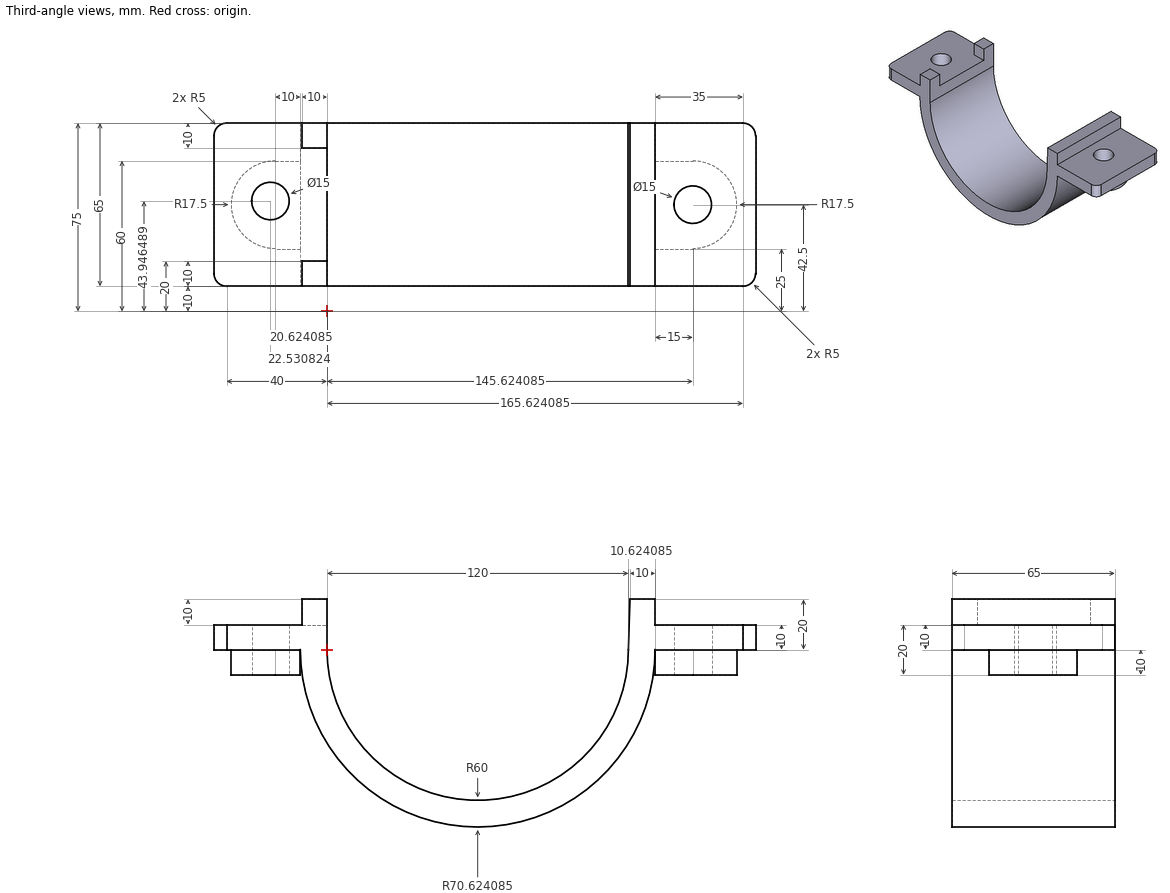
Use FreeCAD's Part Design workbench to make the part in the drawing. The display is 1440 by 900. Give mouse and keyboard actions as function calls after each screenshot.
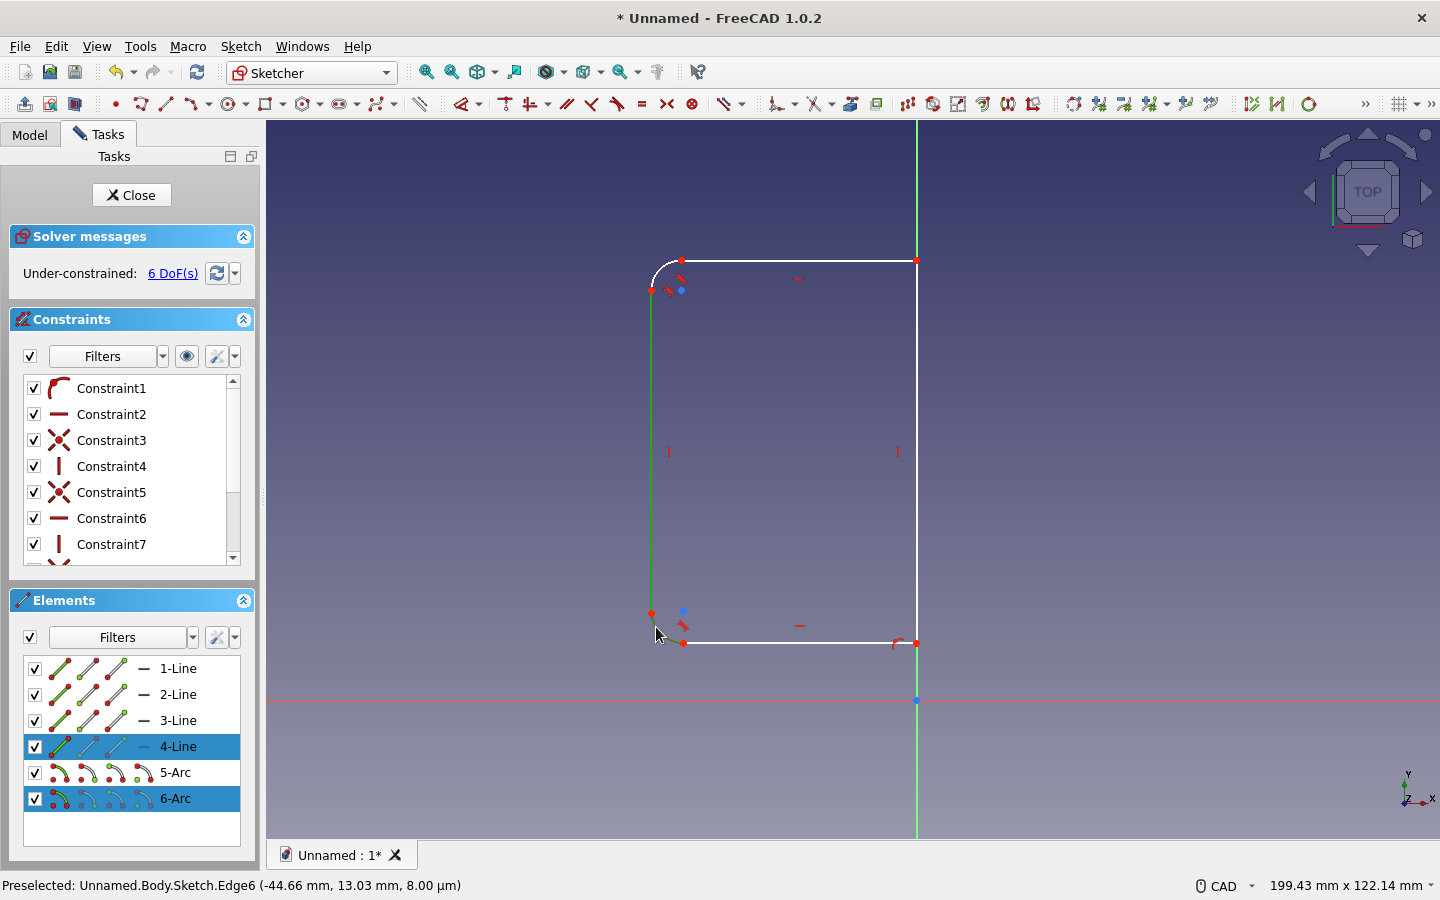
click(617, 104)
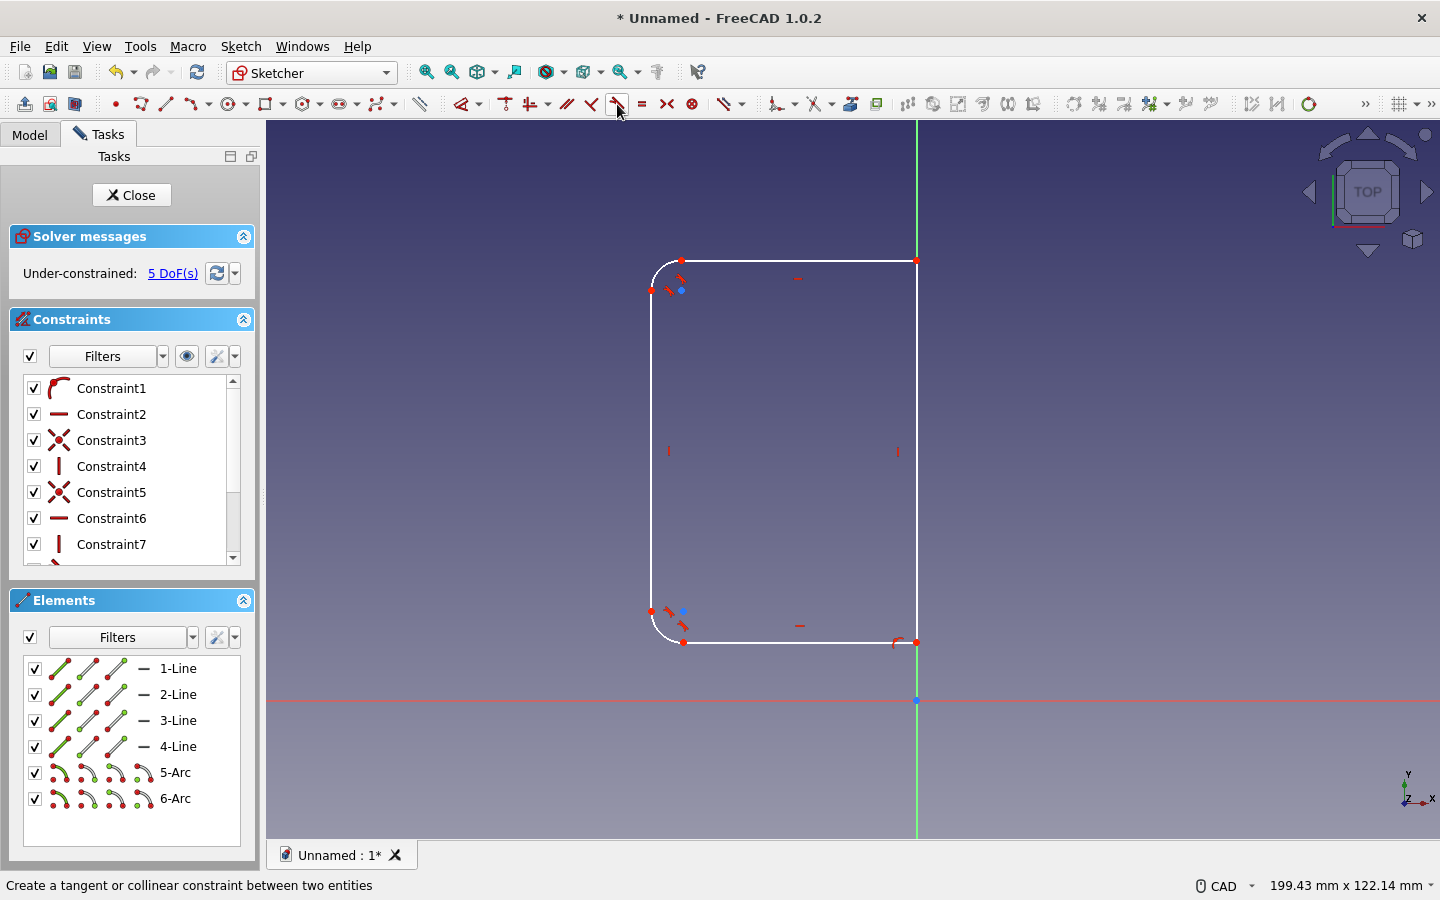
click(668, 264)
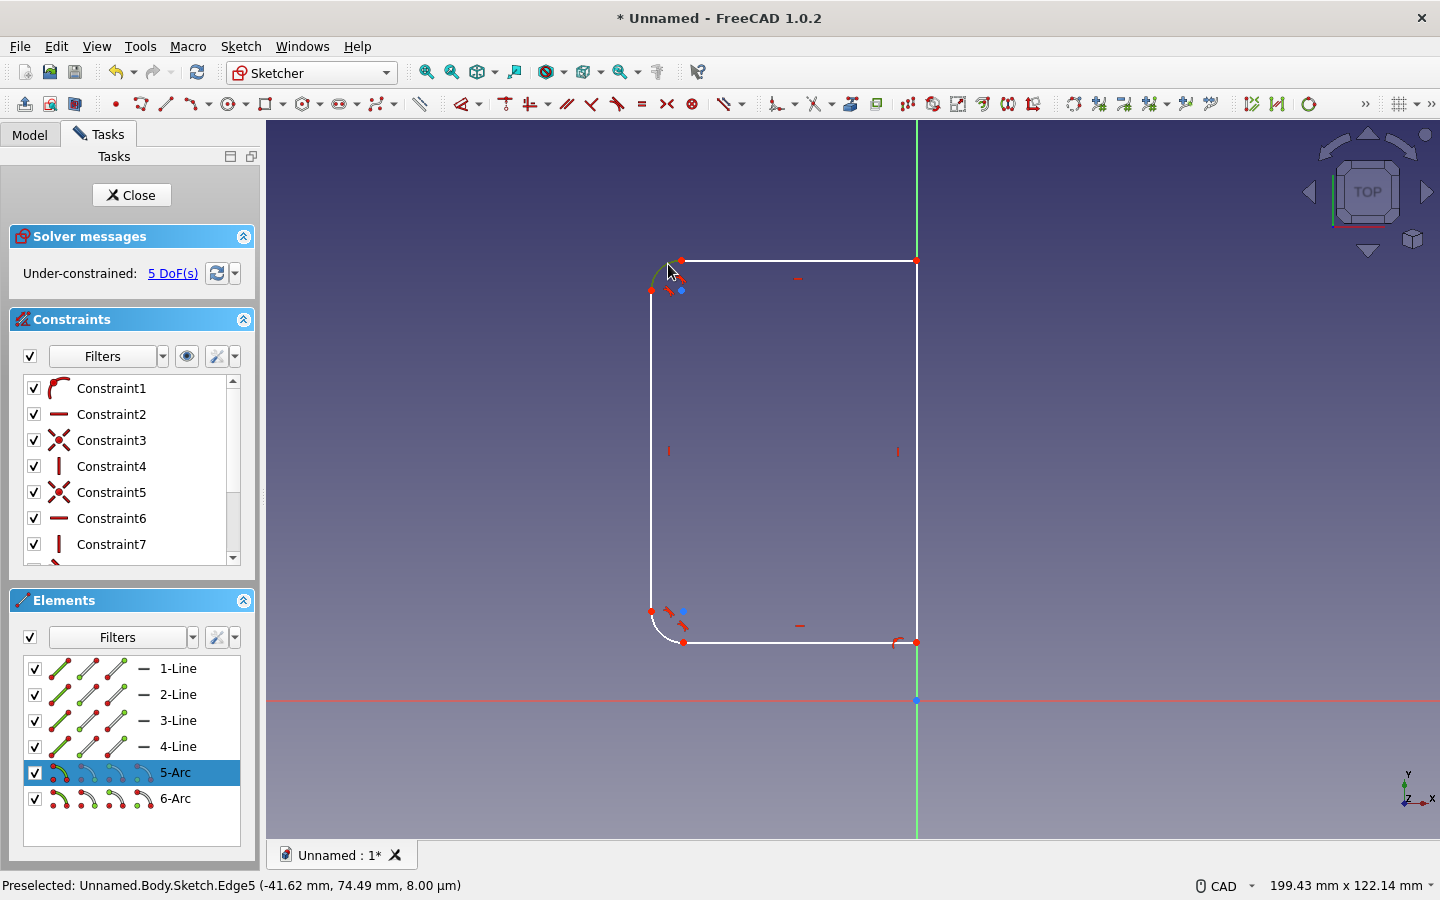
click(655, 626)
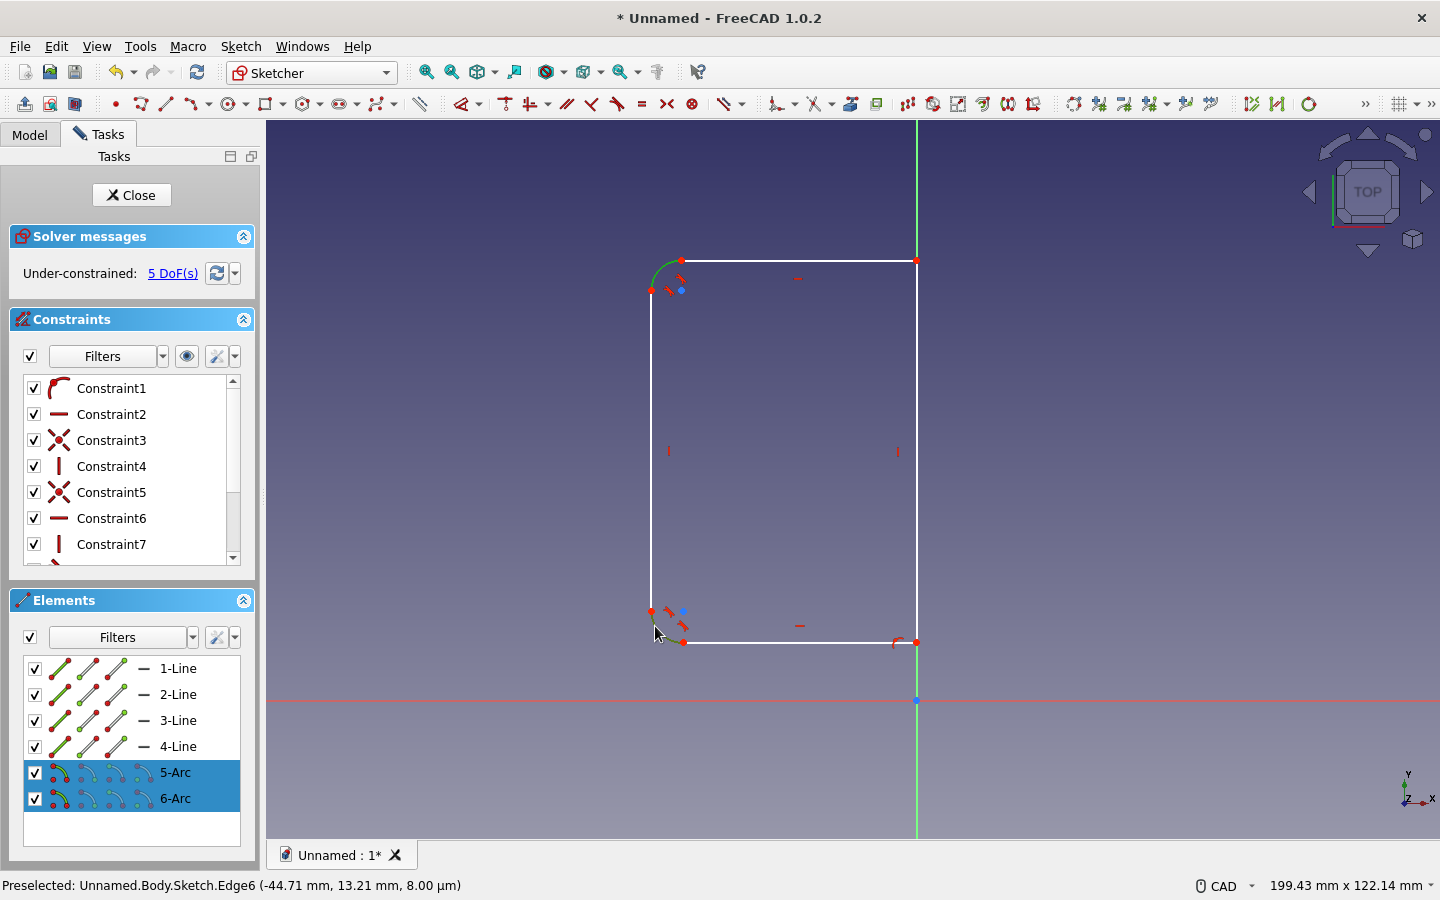
key(e)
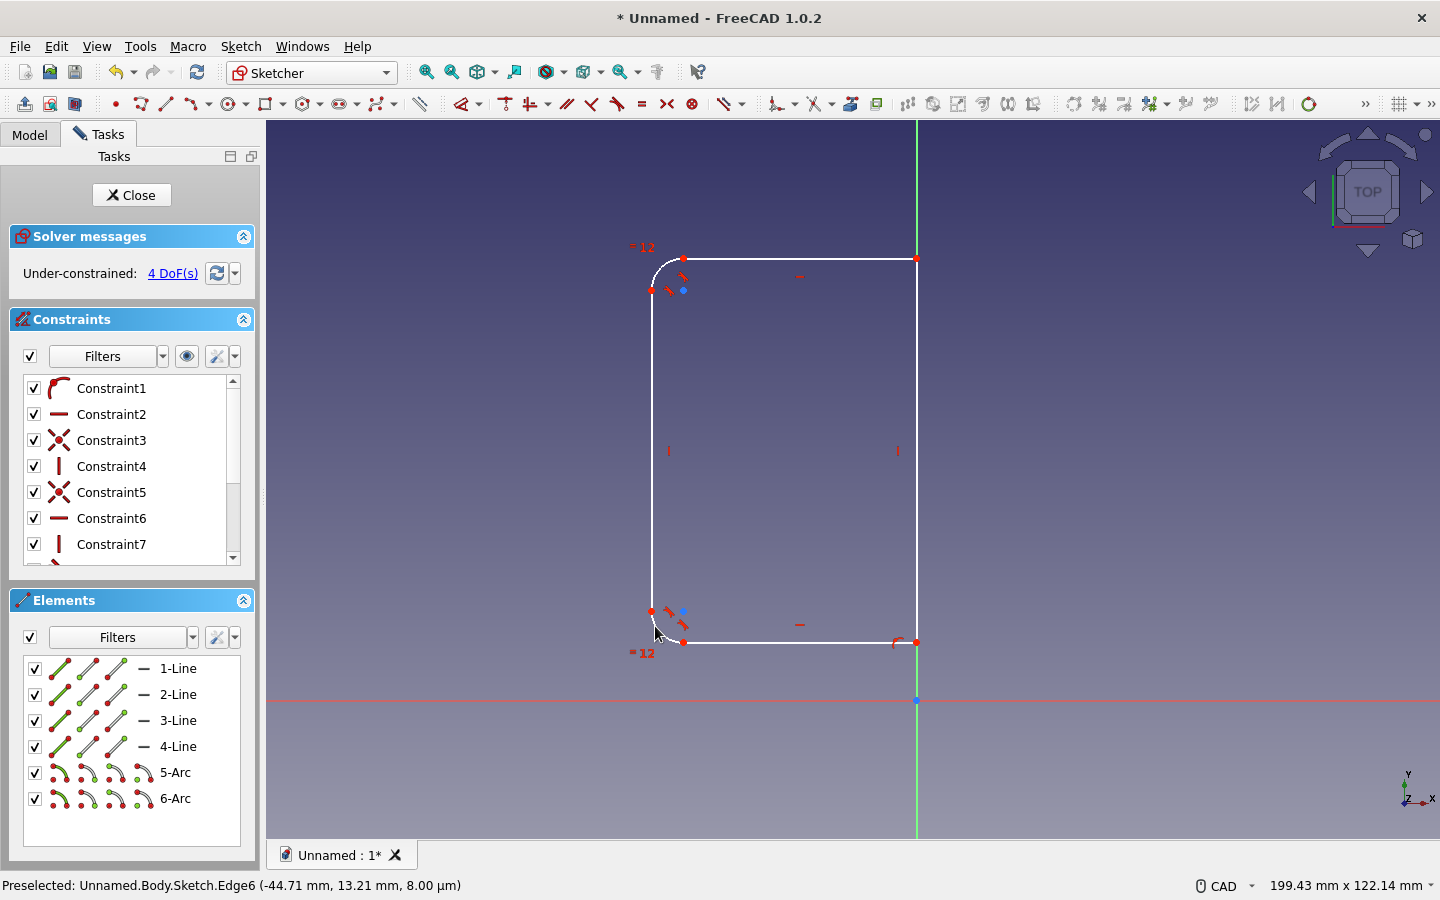
key(d)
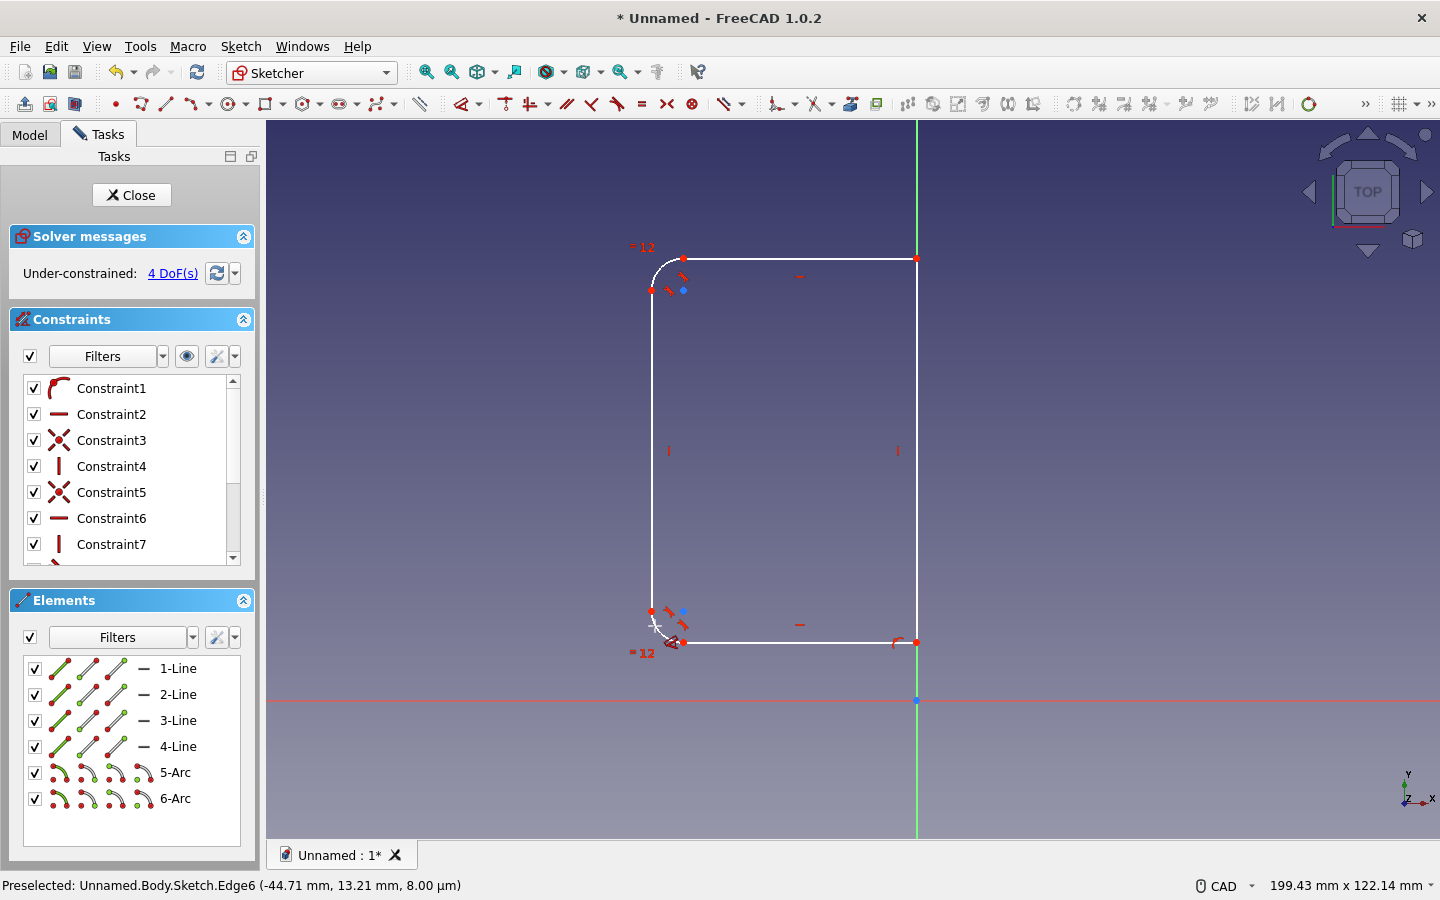
scroll(669, 262, up, 2)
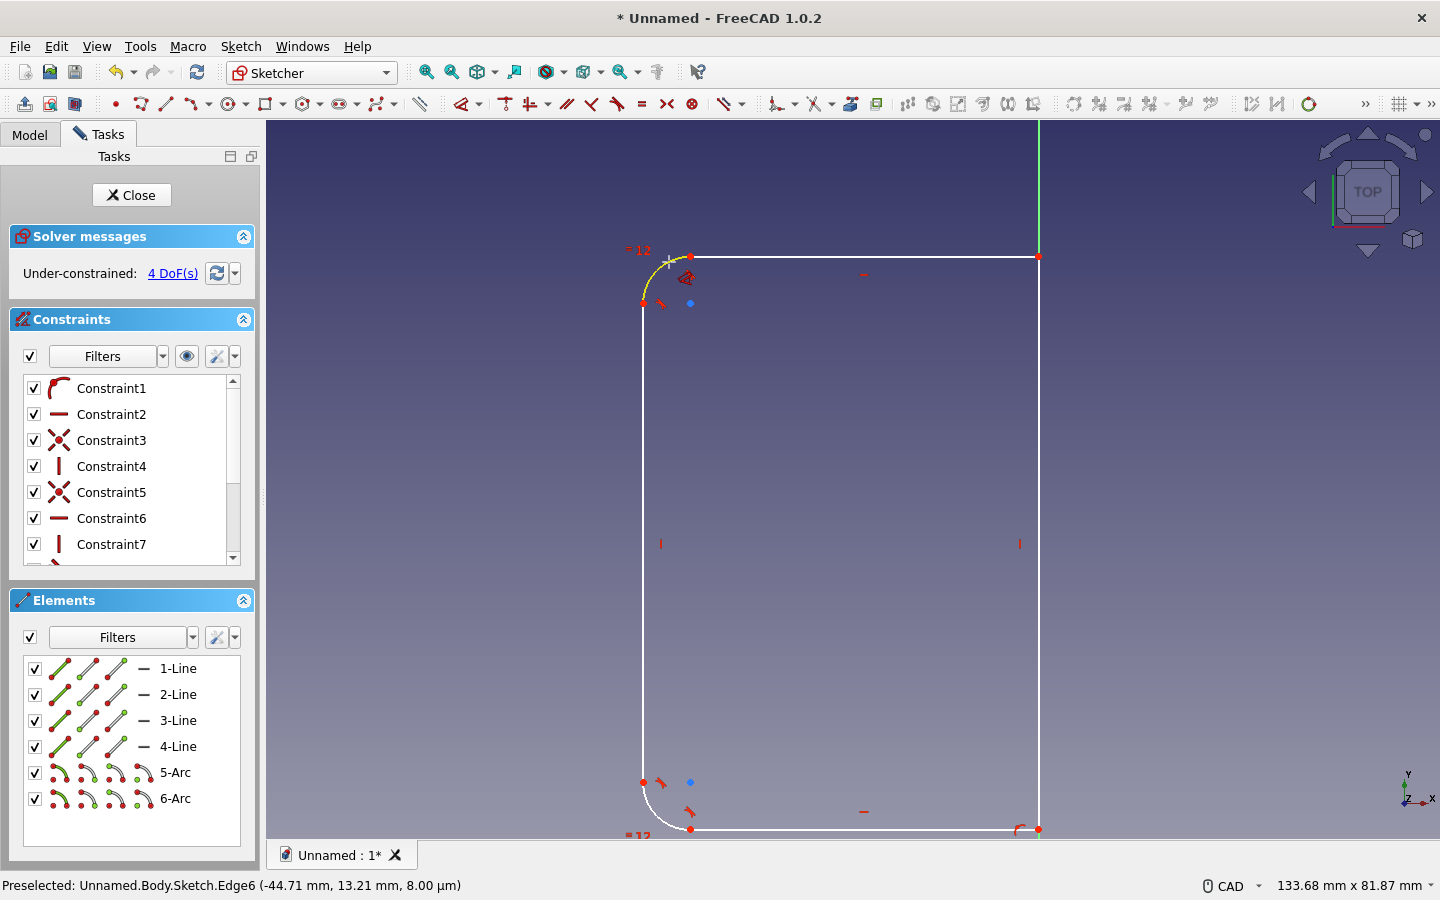
click(669, 262)
click(654, 233)